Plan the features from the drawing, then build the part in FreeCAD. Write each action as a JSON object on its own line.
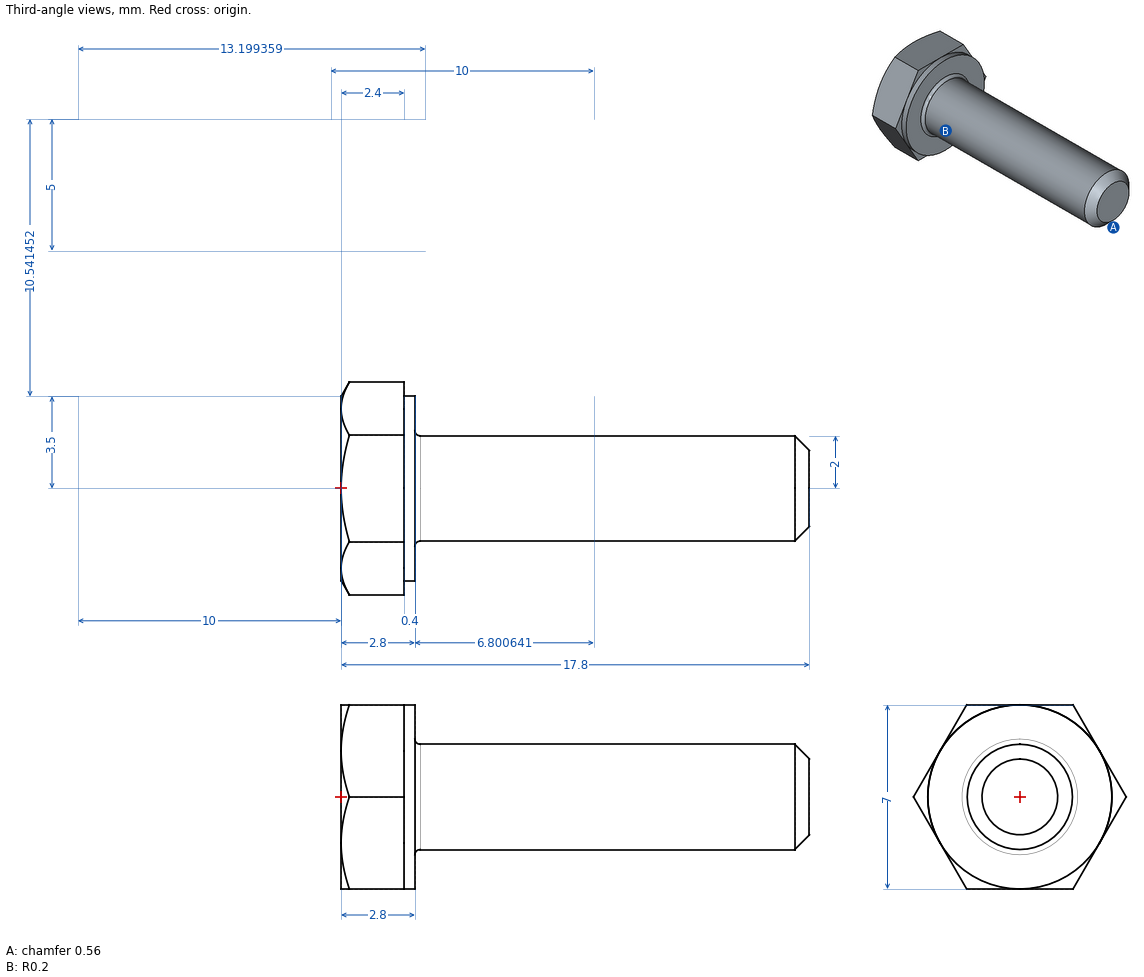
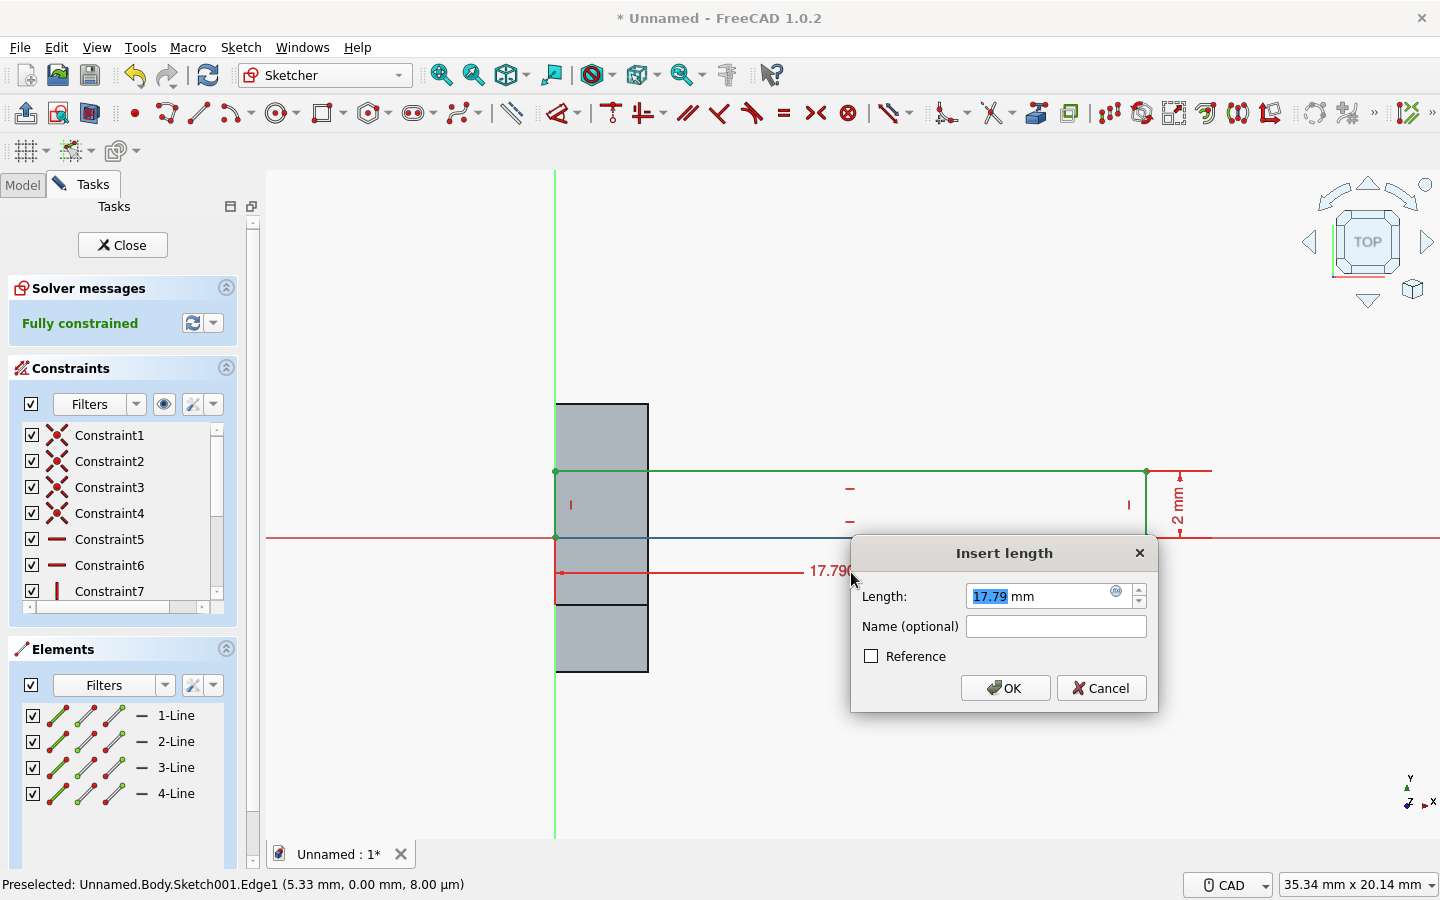
{"action": "type", "text": "17.8"}
{"action": "key", "text": "Return"}
{"action": "key", "text": "Escape"}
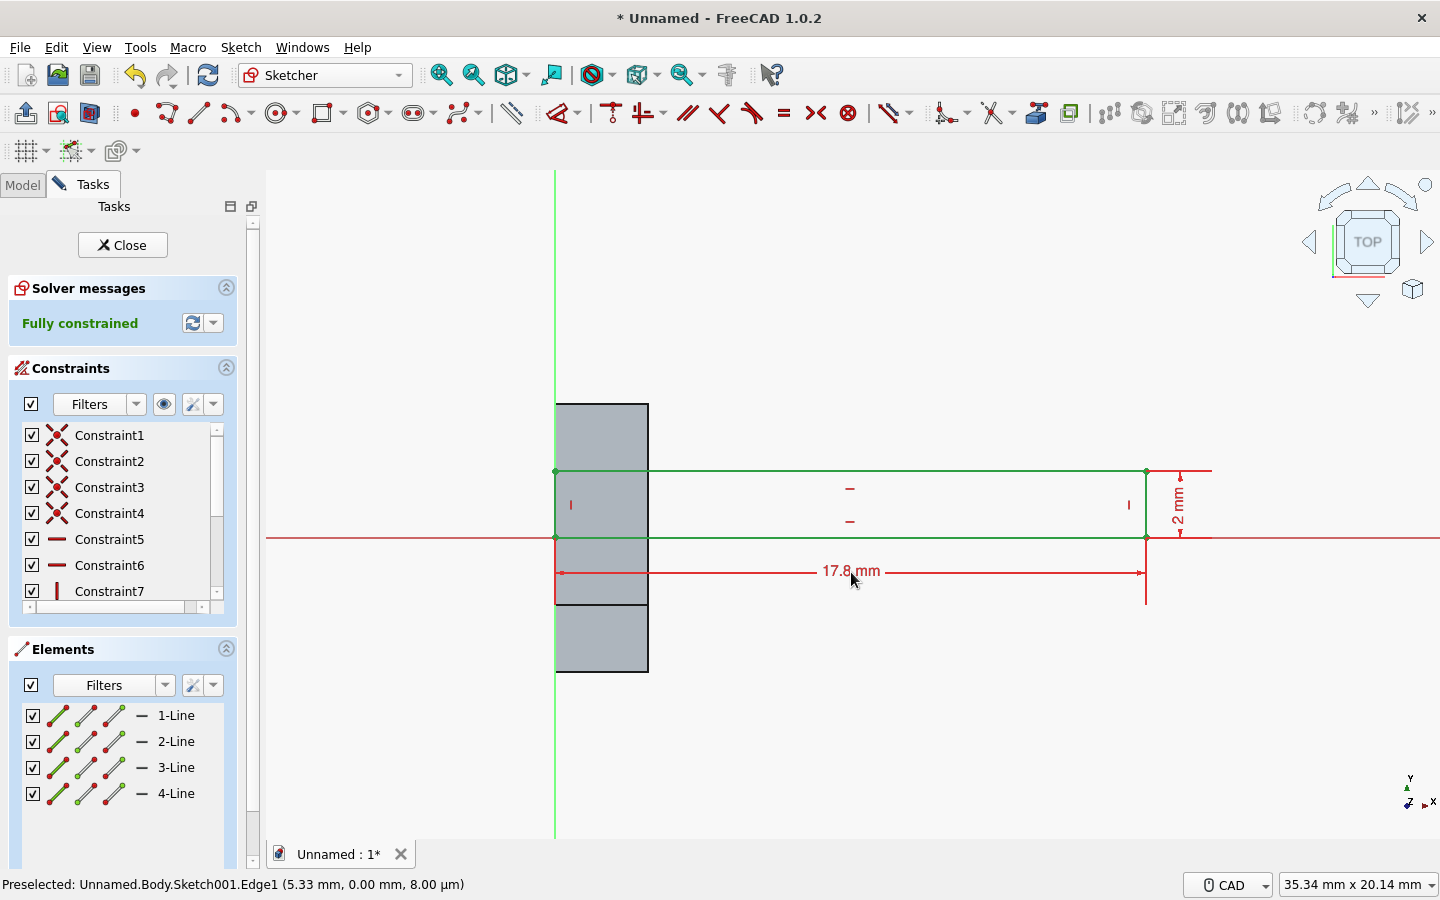
{"action": "left_click", "coordinate": [123, 245]}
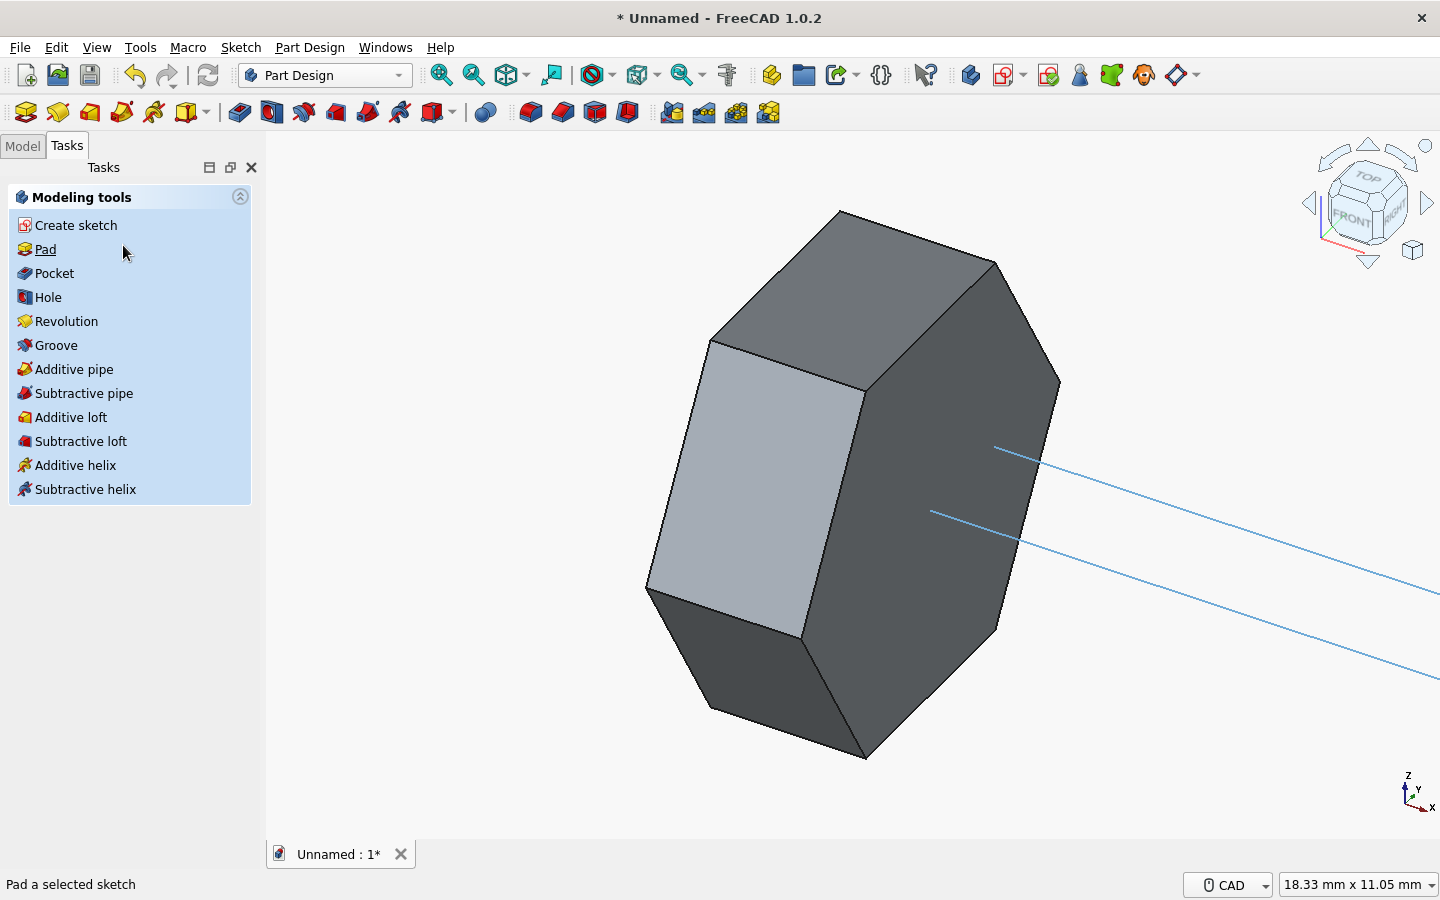
{"action": "left_click", "coordinate": [58, 112]}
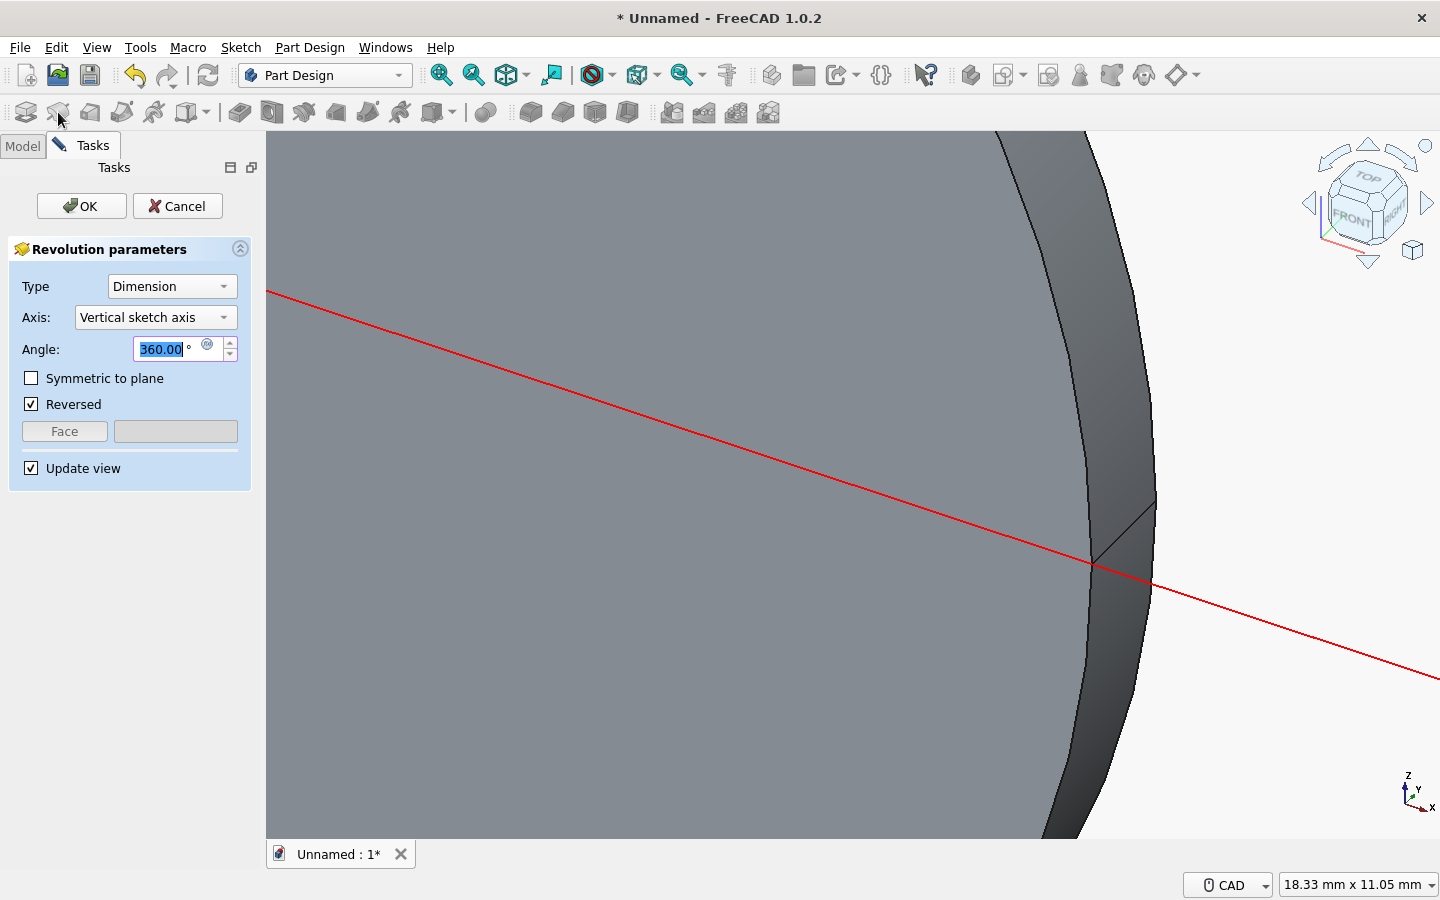
{"action": "left_click", "coordinate": [156, 318]}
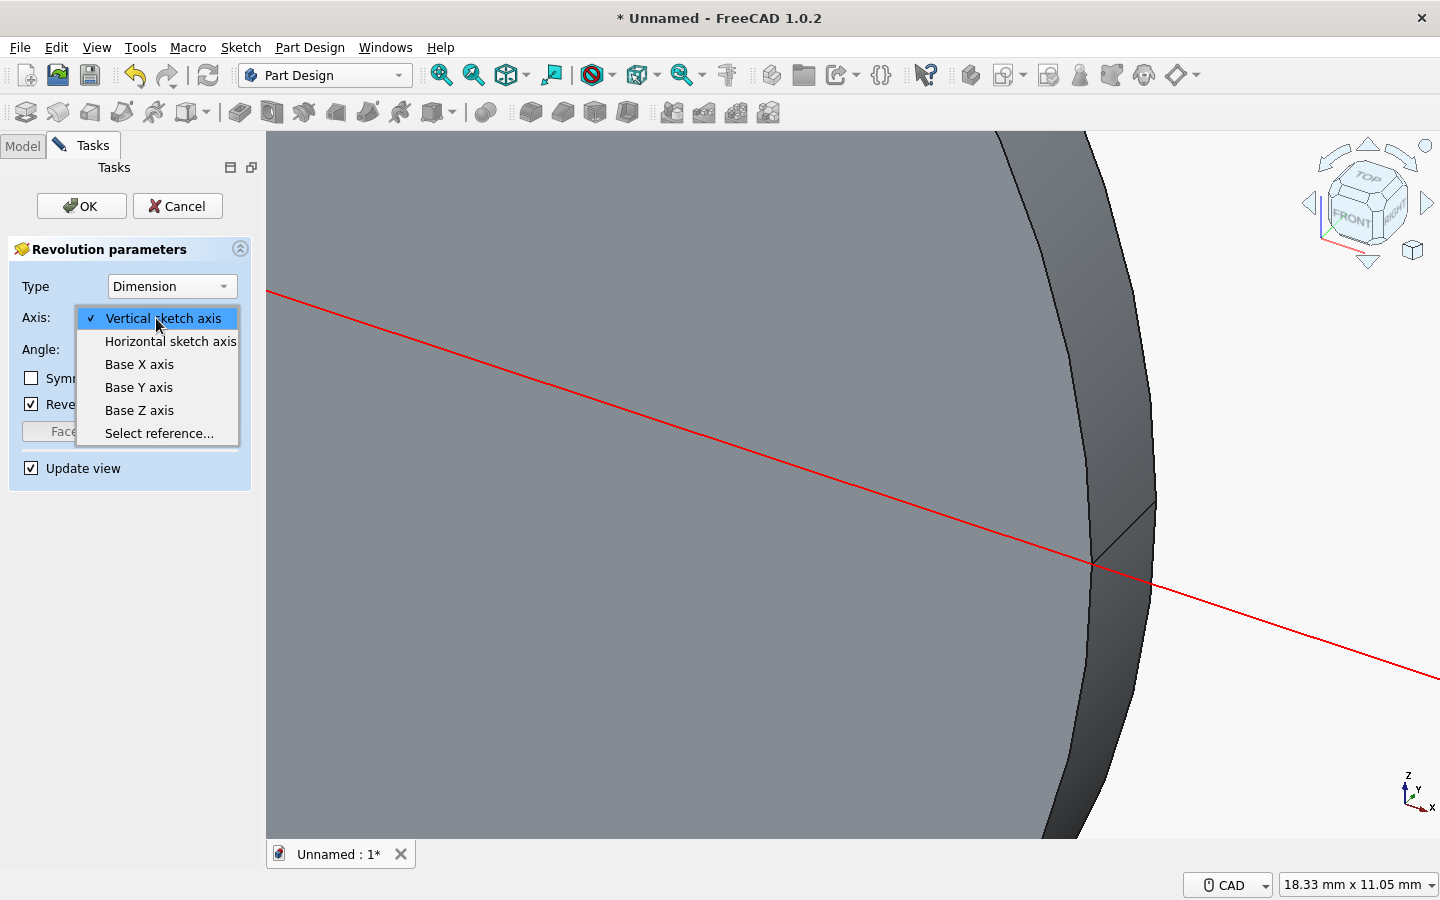
{"action": "left_click", "coordinate": [156, 342]}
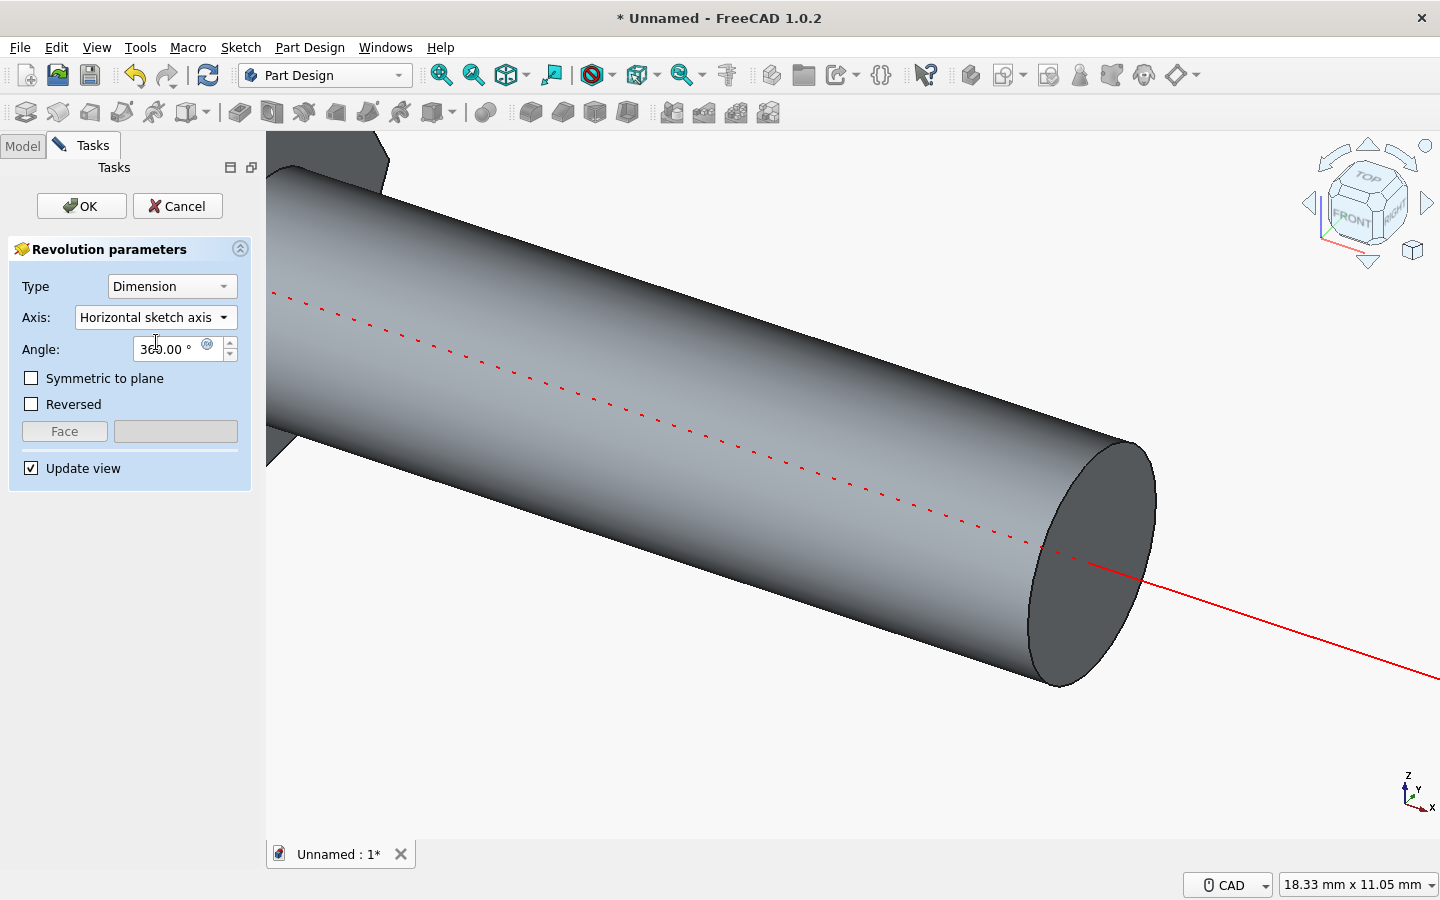
{"action": "left_click", "coordinate": [82, 206]}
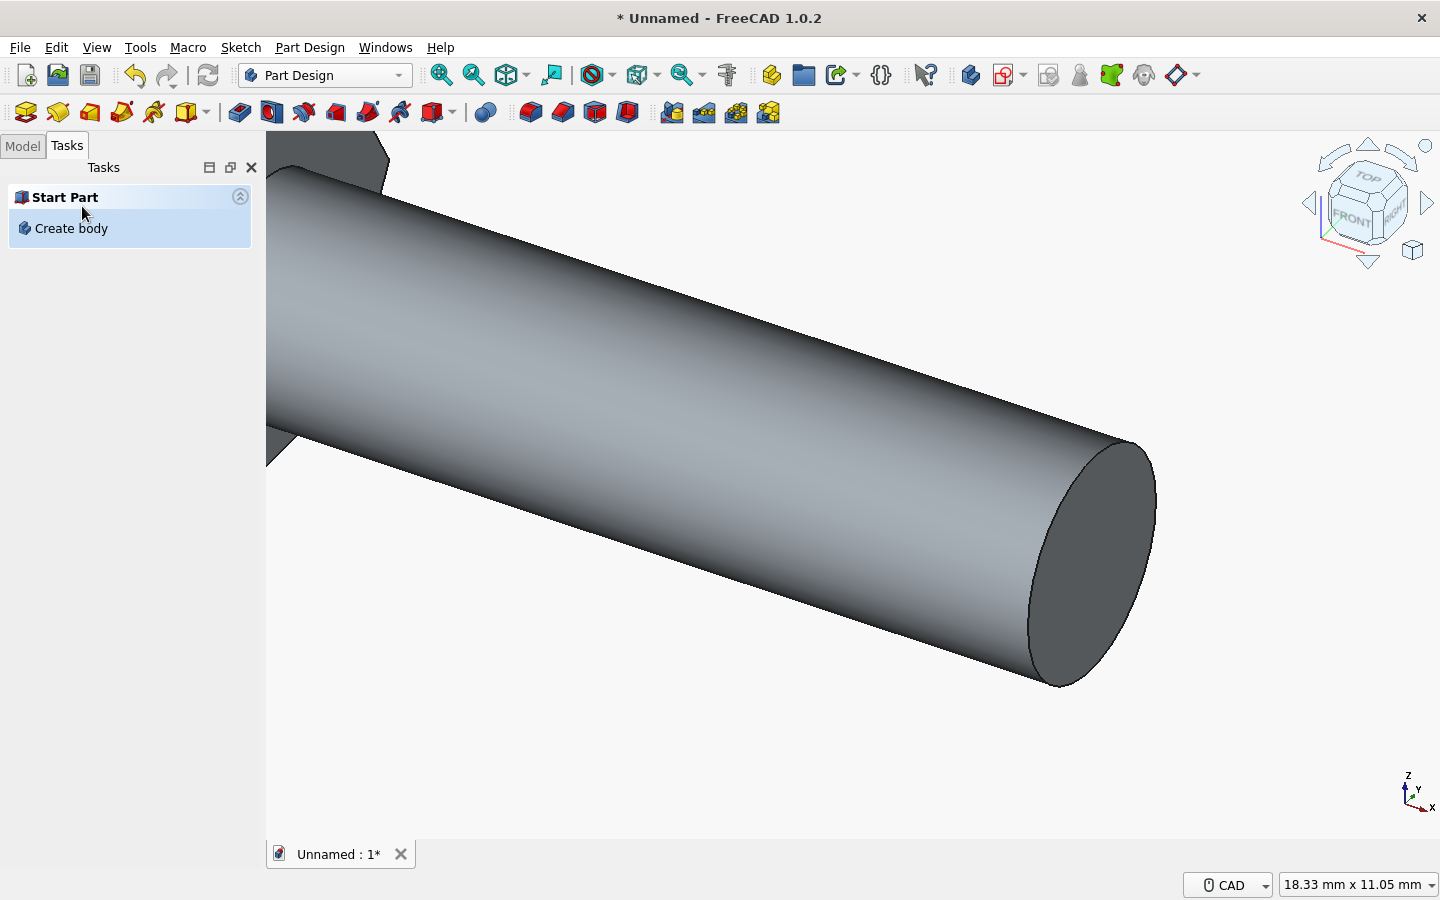
{"action": "key", "text": "v f"}